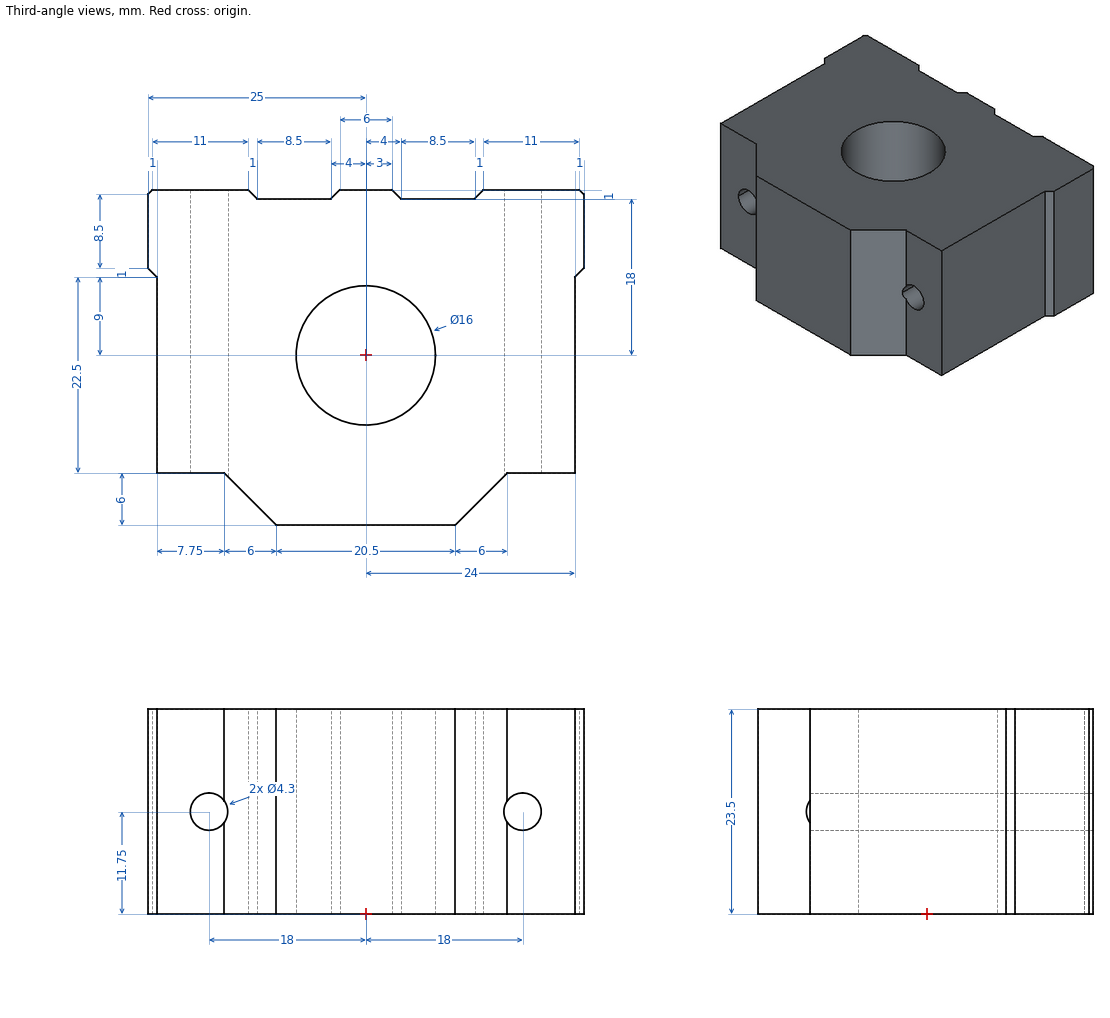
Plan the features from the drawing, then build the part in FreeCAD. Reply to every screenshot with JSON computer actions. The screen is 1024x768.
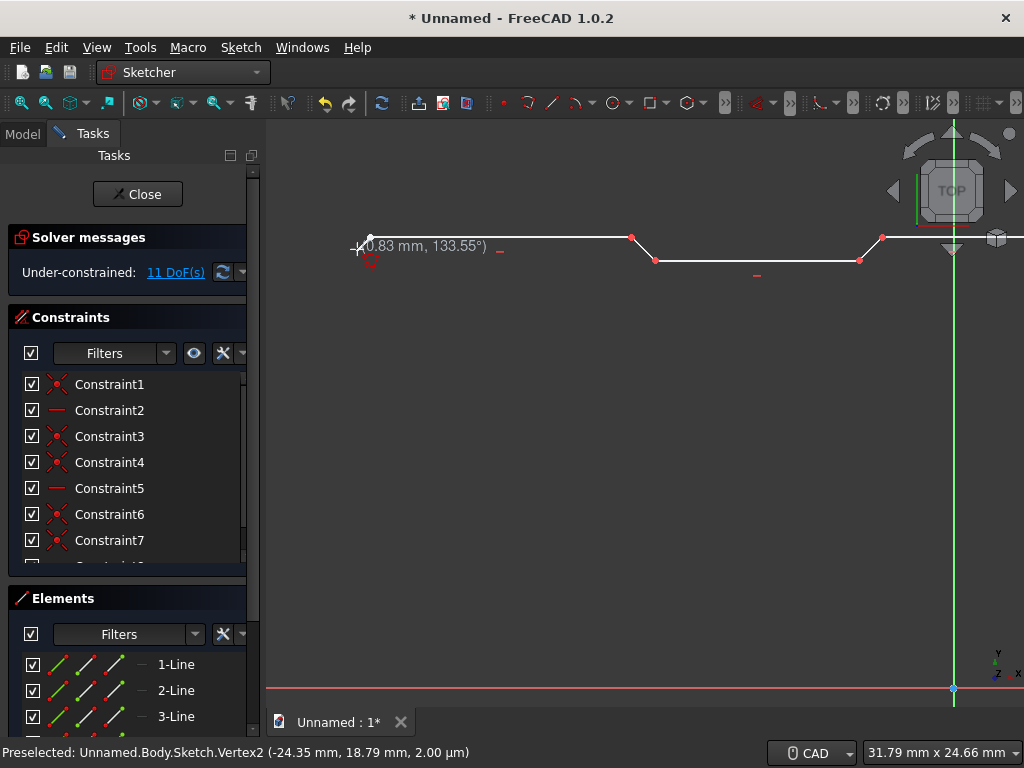
{"action": "left_click", "coordinate": [358, 247]}
{"action": "left_click", "coordinate": [358, 450]}
{"action": "left_click", "coordinate": [382, 474]}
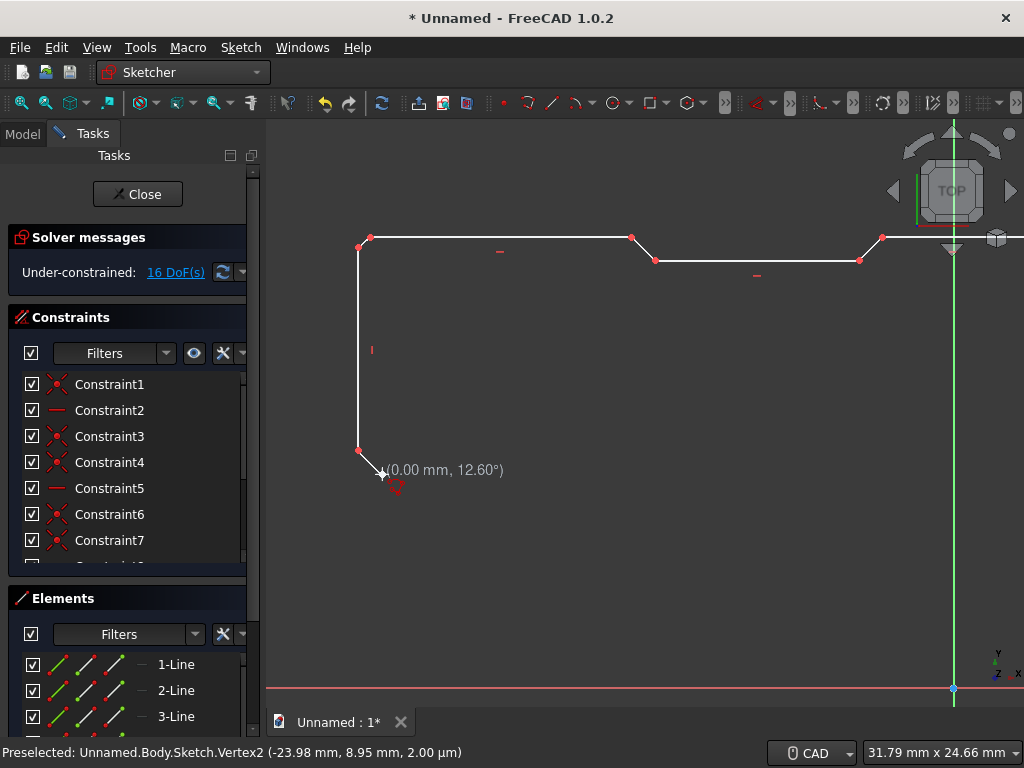
{"action": "scroll", "coordinate": [357, 249], "scroll_direction": "down", "scroll_amount": 5}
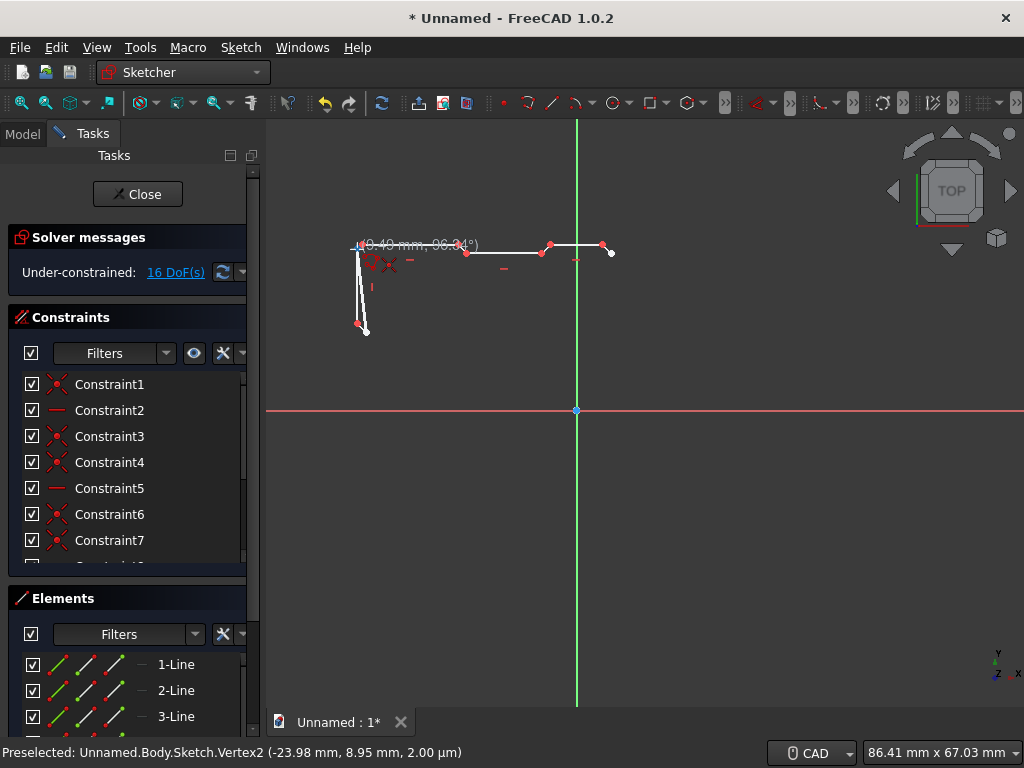
{"action": "left_click", "coordinate": [366, 529]}
{"action": "left_click", "coordinate": [434, 529]}
{"action": "left_click", "coordinate": [487, 582]}
{"action": "left_click", "coordinate": [667, 582]}
{"action": "left_click", "coordinate": [719, 529]}
{"action": "left_click", "coordinate": [787, 529]}
{"action": "left_click", "coordinate": [787, 332]}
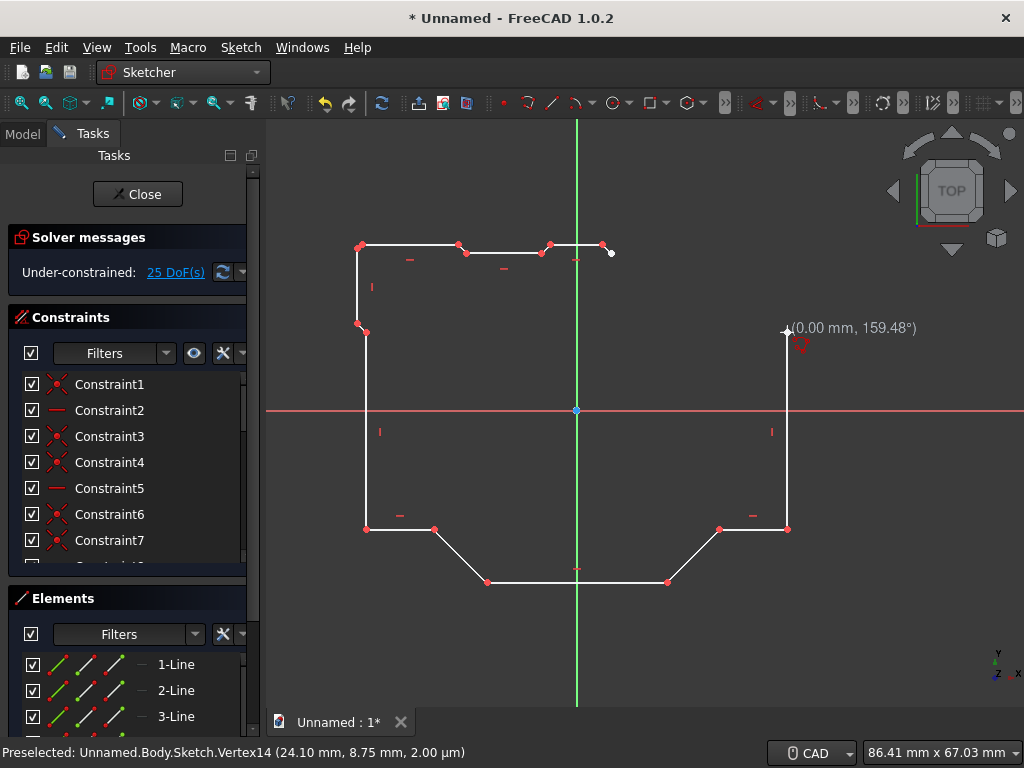
{"action": "scroll", "coordinate": [796, 323], "scroll_direction": "up", "scroll_amount": 2}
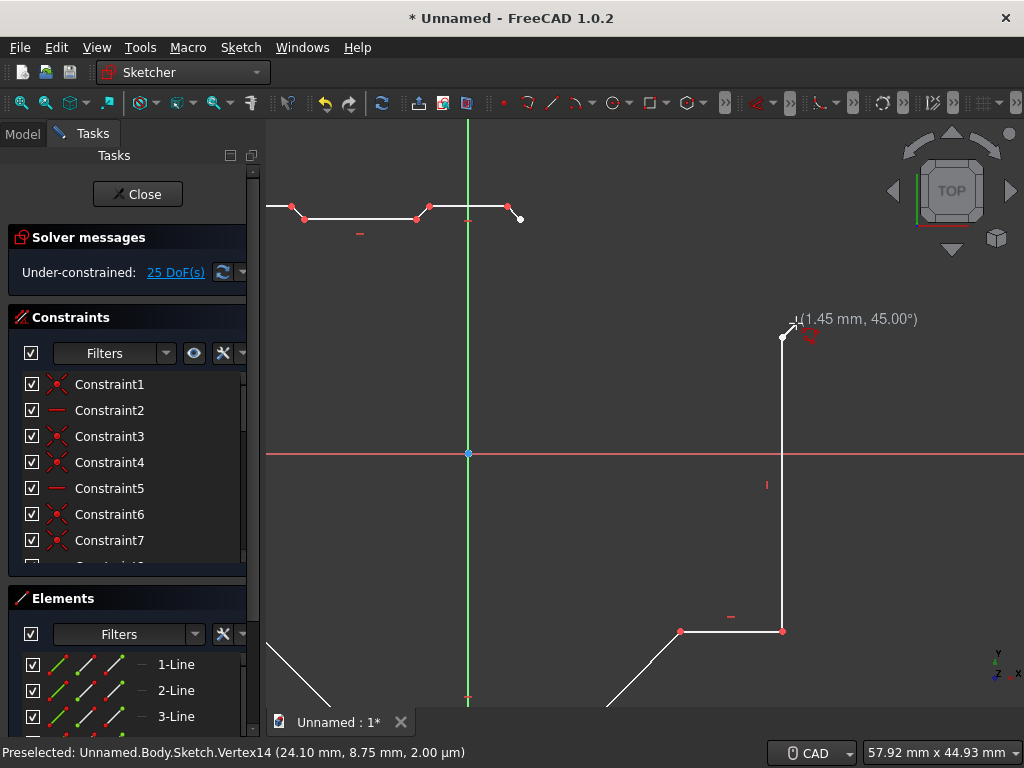
{"action": "left_click", "coordinate": [796, 323]}
{"action": "left_click", "coordinate": [796, 212]}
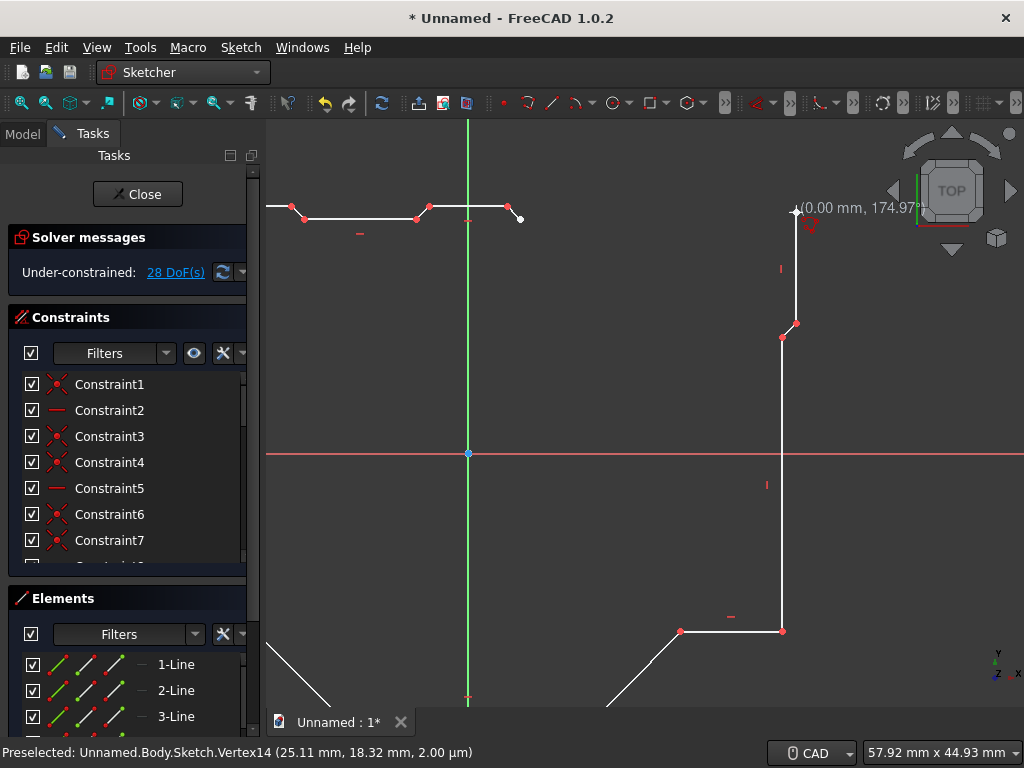
{"action": "scroll", "coordinate": [789, 205], "scroll_direction": "up", "scroll_amount": 3}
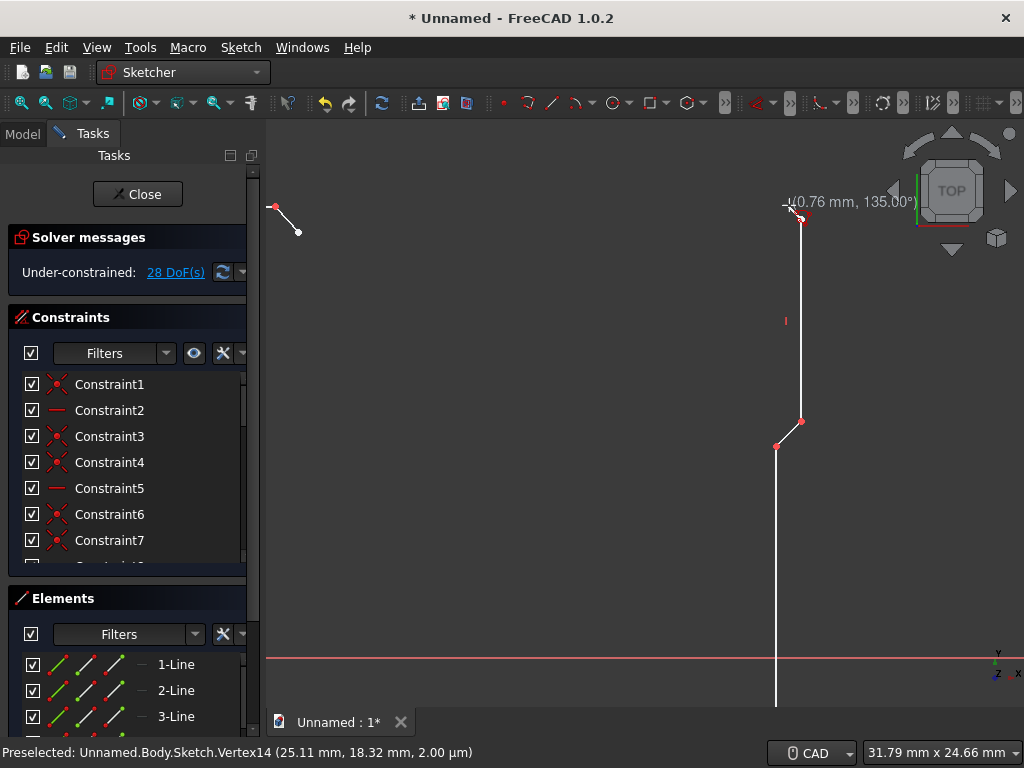
{"action": "left_click", "coordinate": [788, 205]}
{"action": "left_click", "coordinate": [526, 205]}
{"action": "left_click", "coordinate": [502, 229]}
{"action": "left_click", "coordinate": [299, 232]}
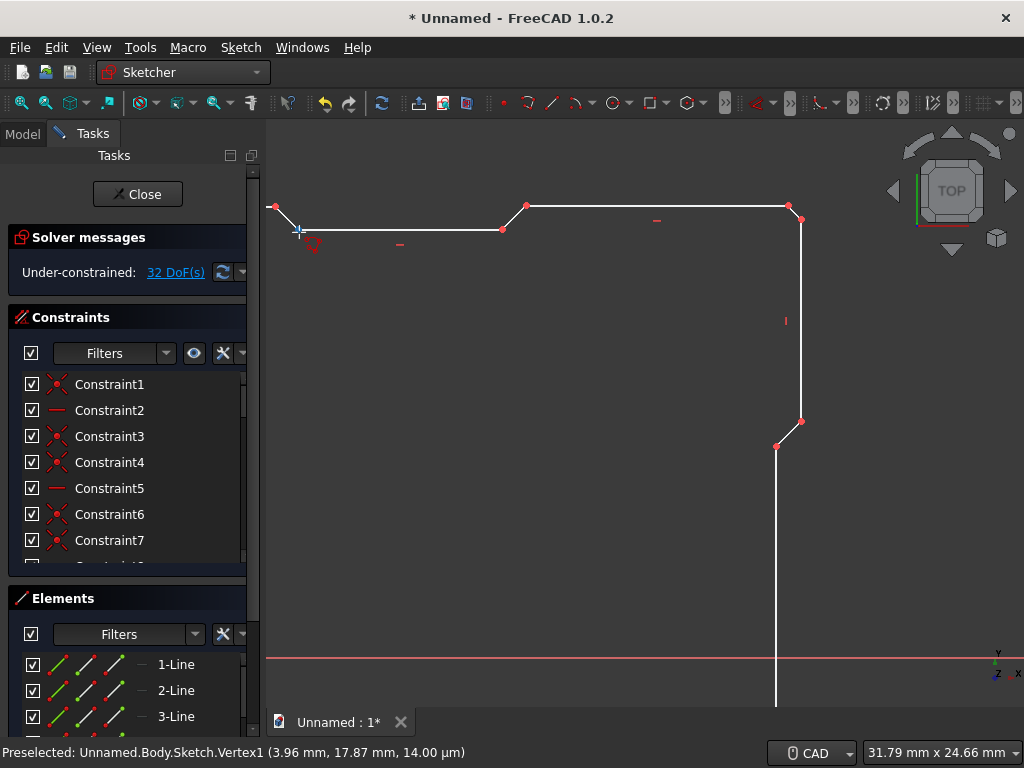
{"action": "left_click", "coordinate": [614, 104]}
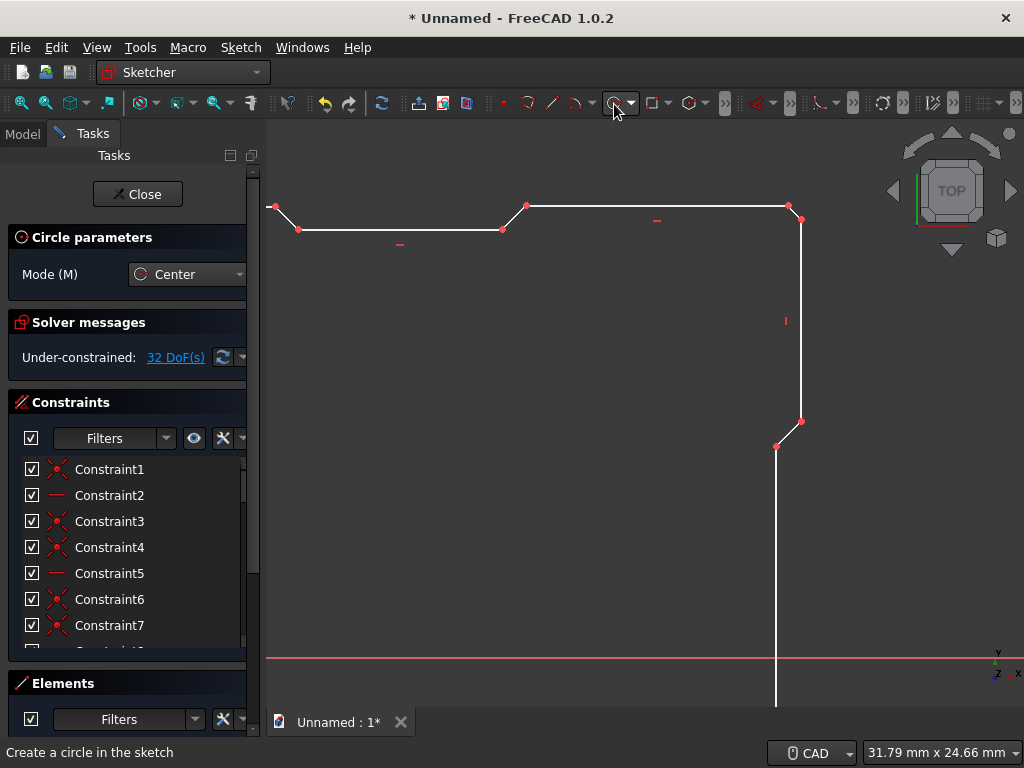
{"action": "scroll", "coordinate": [793, 267], "scroll_direction": "down", "scroll_amount": 5}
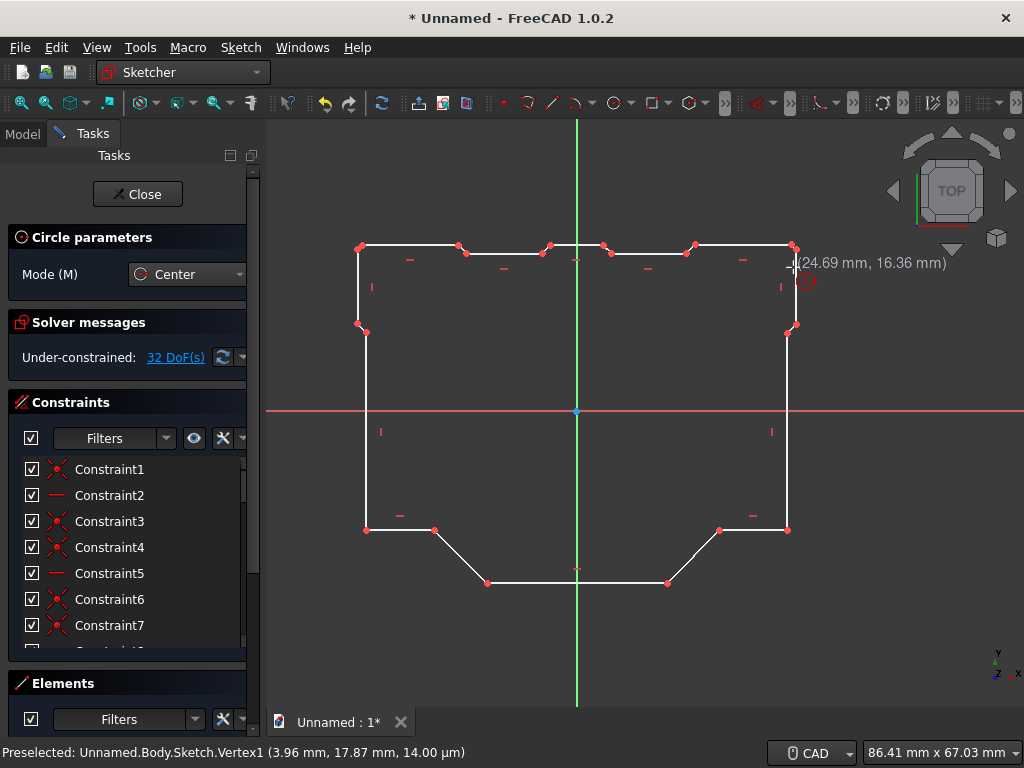
{"action": "left_click", "coordinate": [577, 411]}
{"action": "mouse_move", "coordinate": [626, 361]}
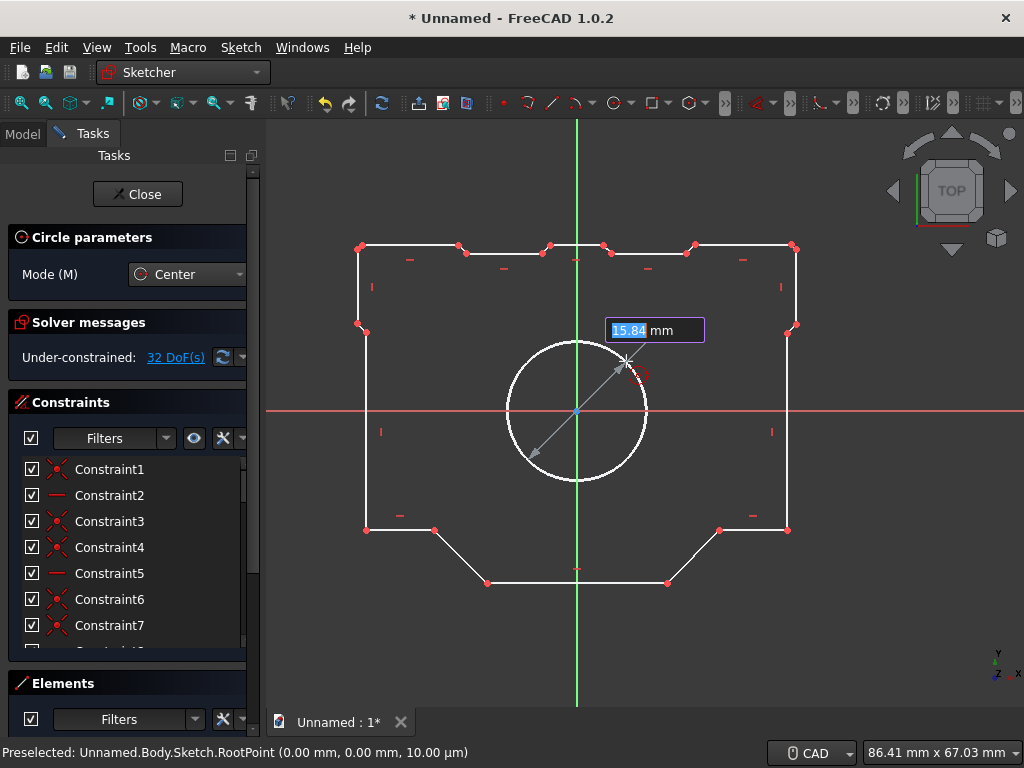
{"action": "type", "text": "16"}
{"action": "key", "text": "Return"}
{"action": "key", "text": "Escape"}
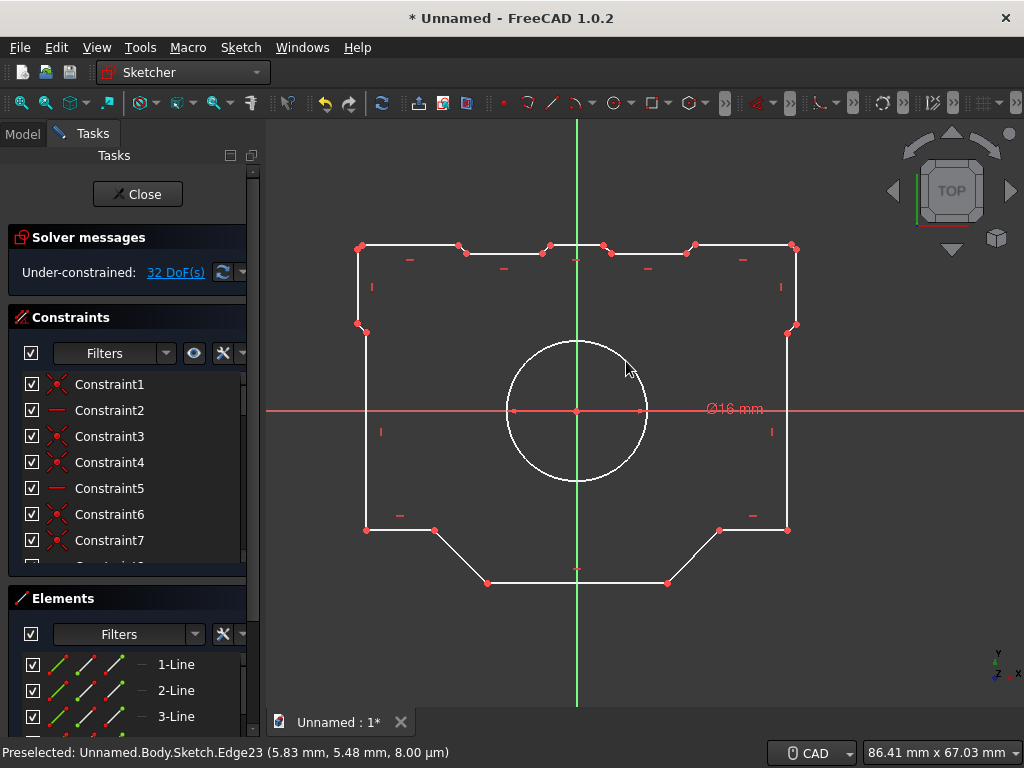
{"action": "left_click", "coordinate": [756, 104]}